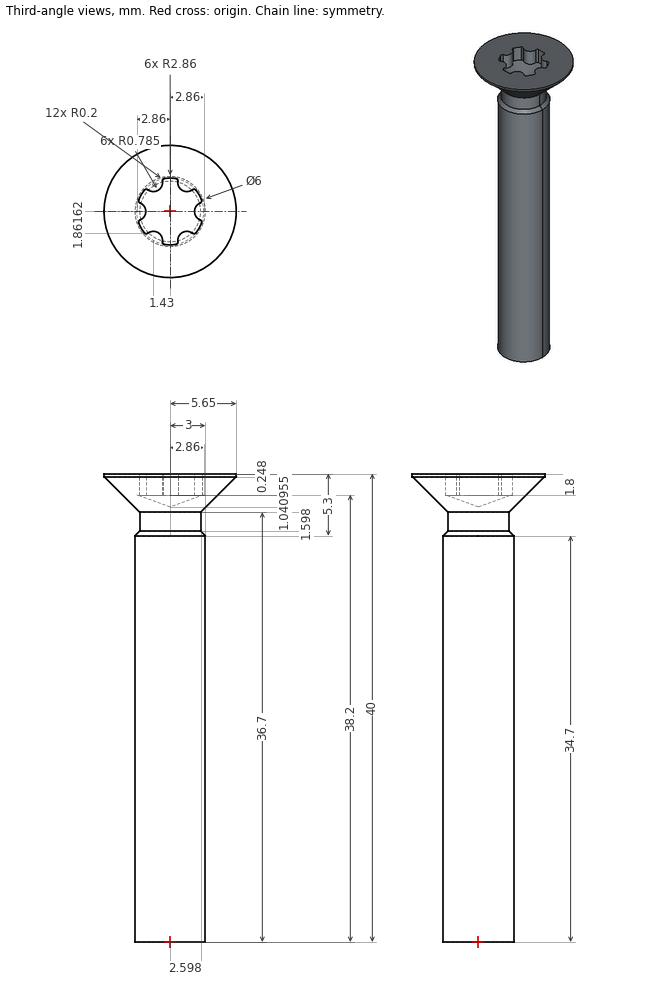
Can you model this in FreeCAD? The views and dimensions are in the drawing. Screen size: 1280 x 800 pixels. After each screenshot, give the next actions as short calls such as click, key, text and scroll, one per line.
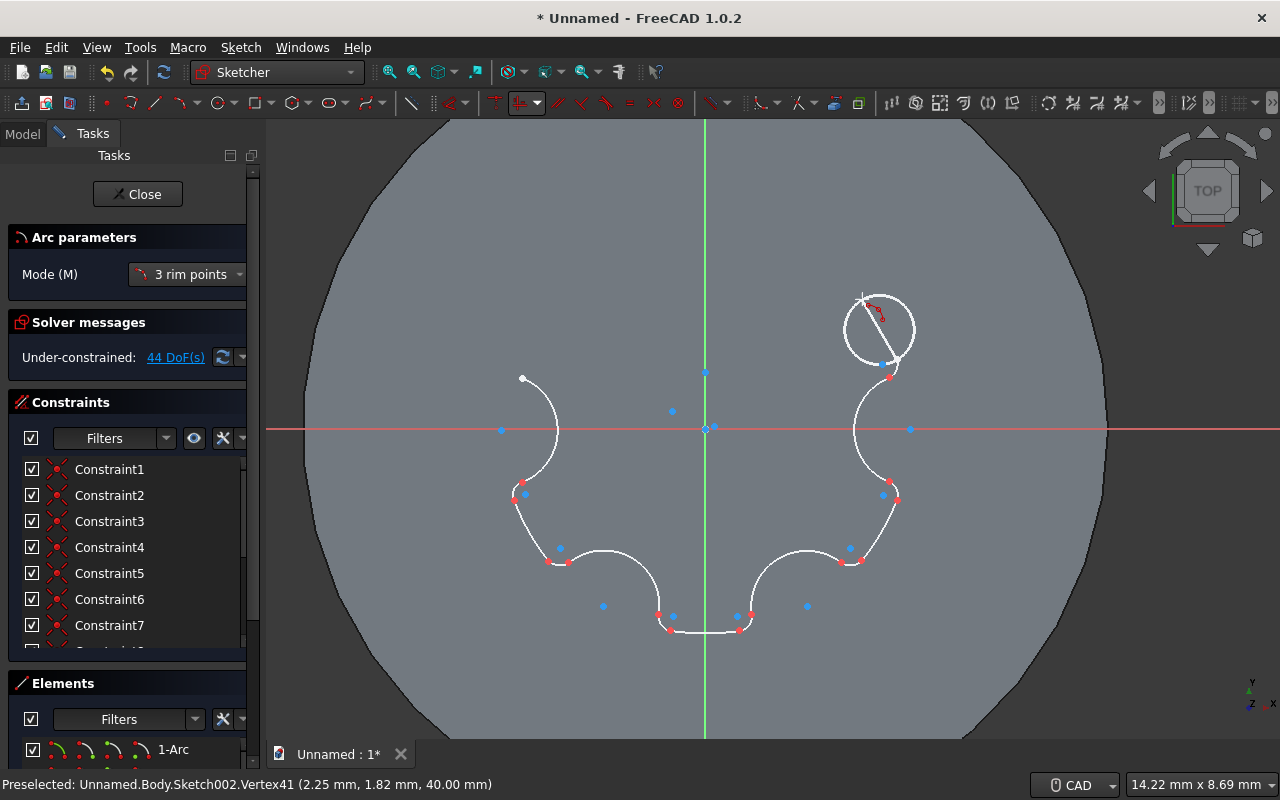
scroll(882, 327, up, 9)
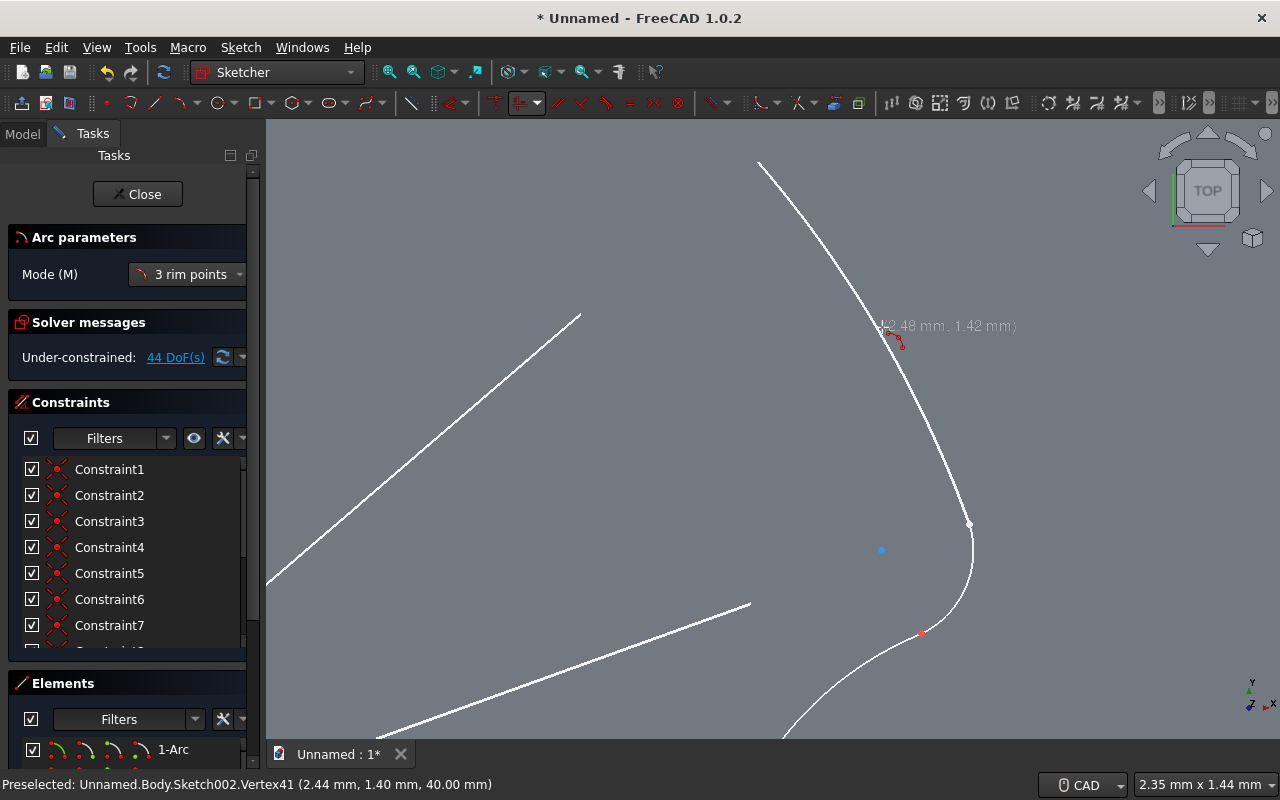
click(878, 327)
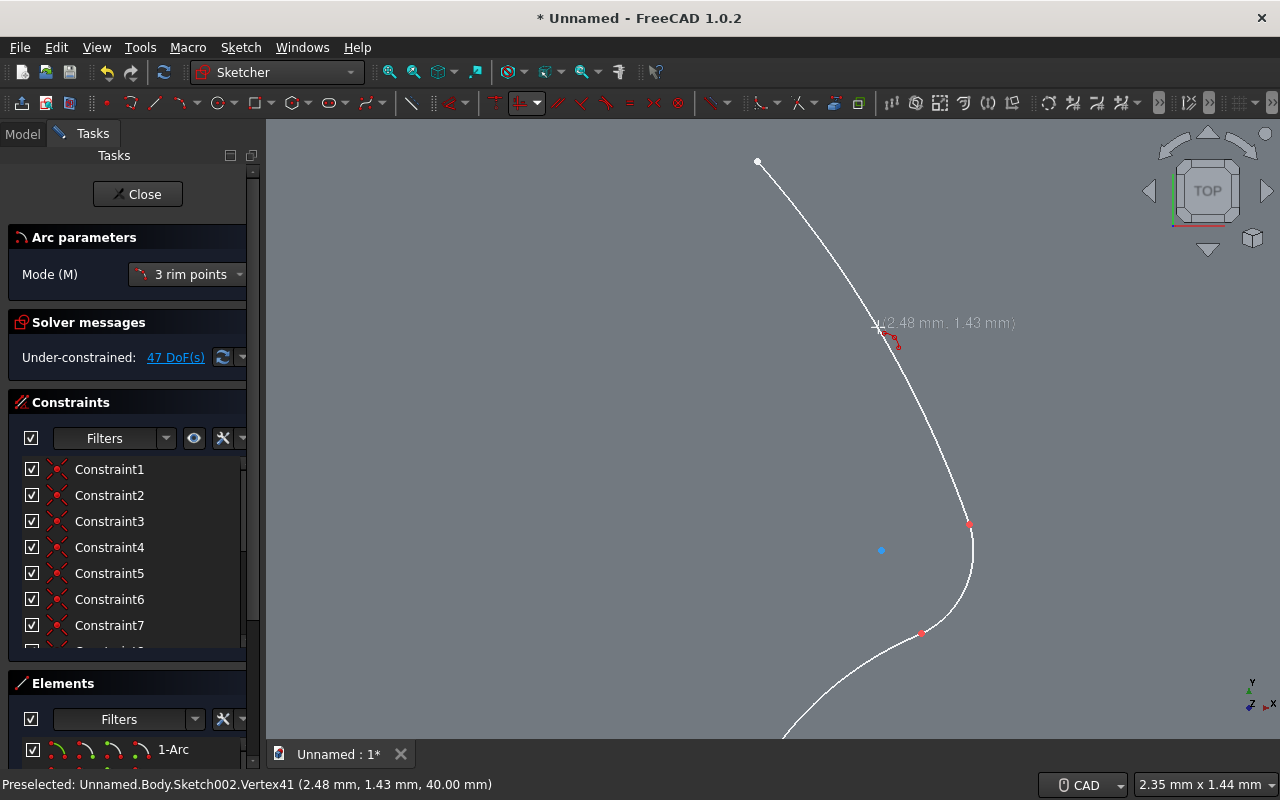
scroll(882, 327, down, 9)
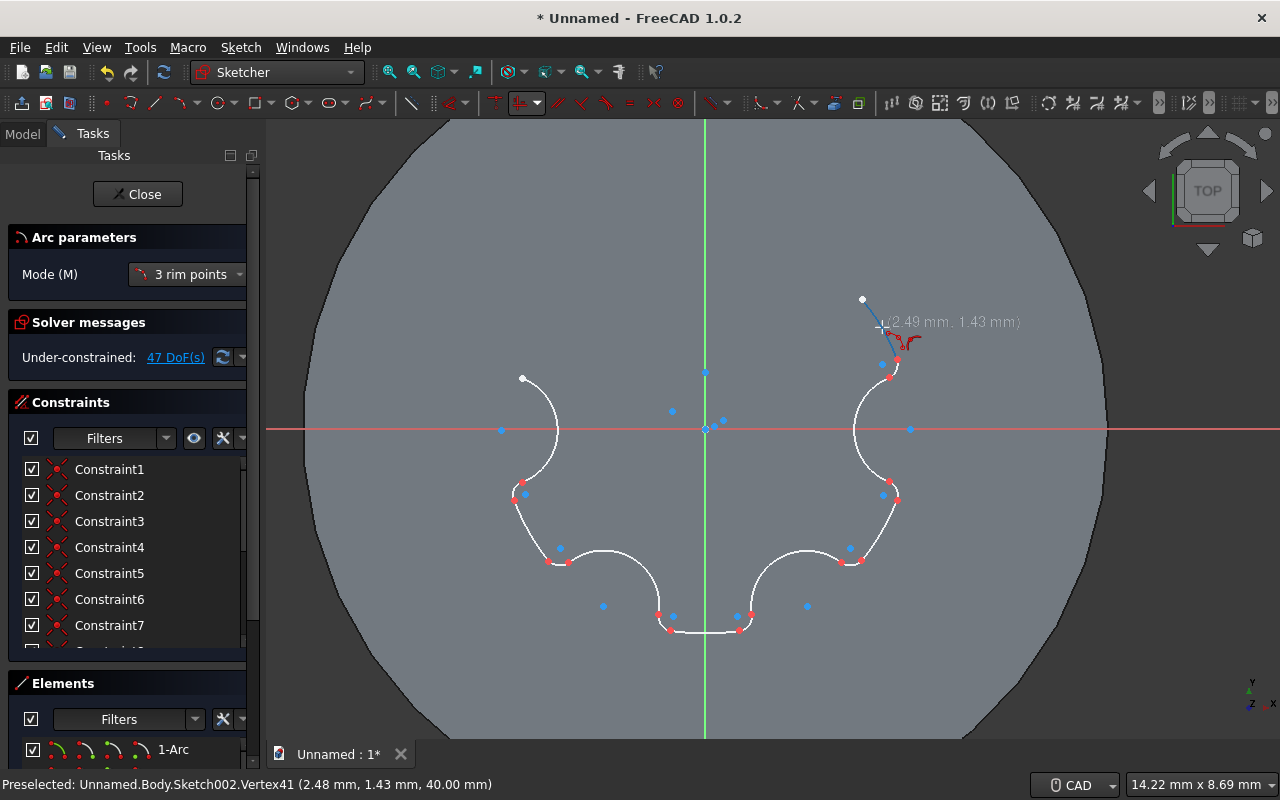
click(862, 300)
click(842, 297)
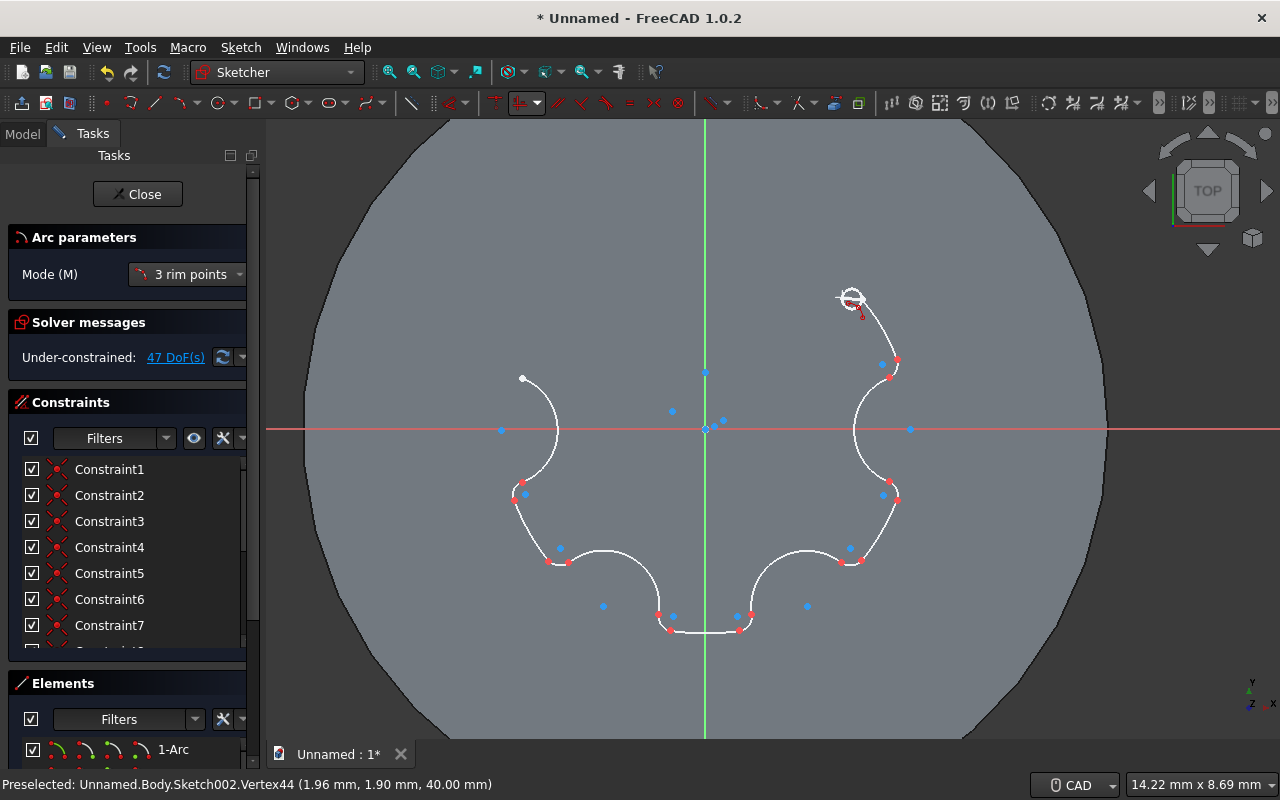
scroll(852, 294, up, 7)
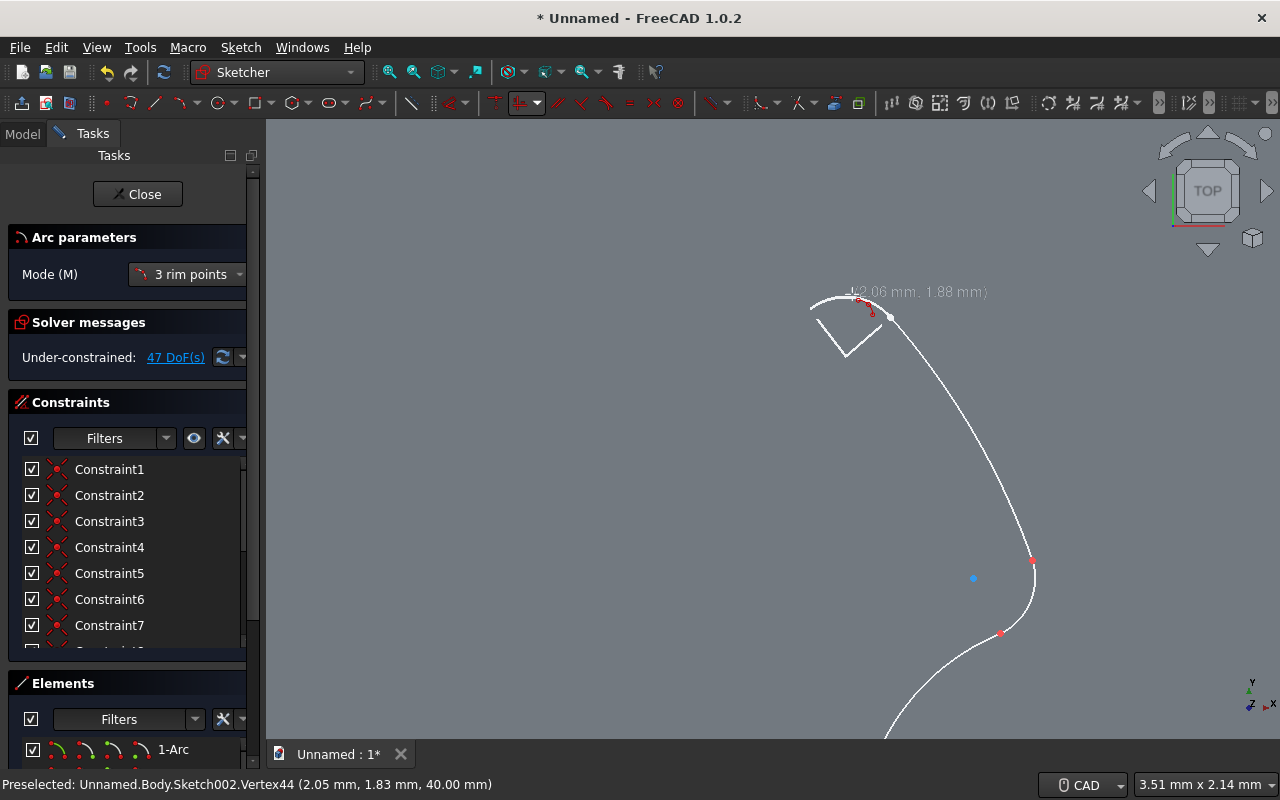
click(852, 291)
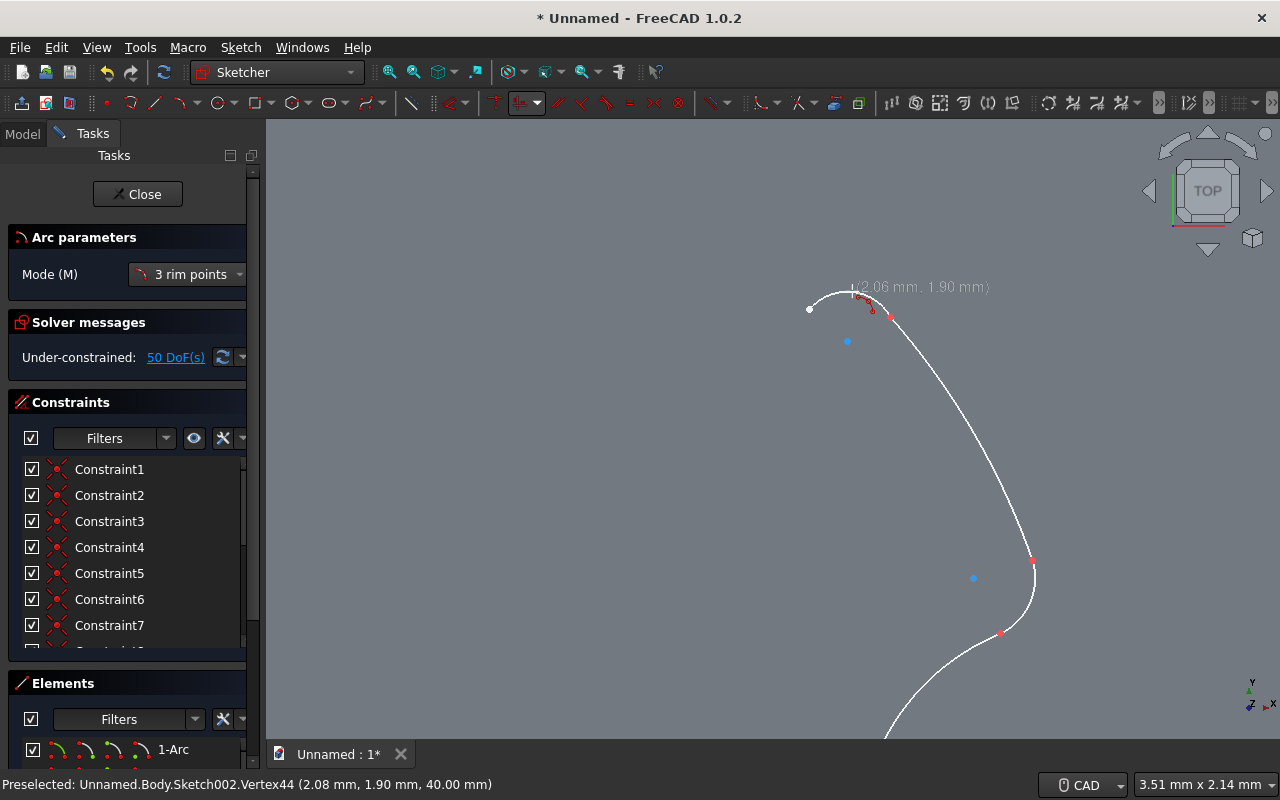
scroll(852, 294, down, 7)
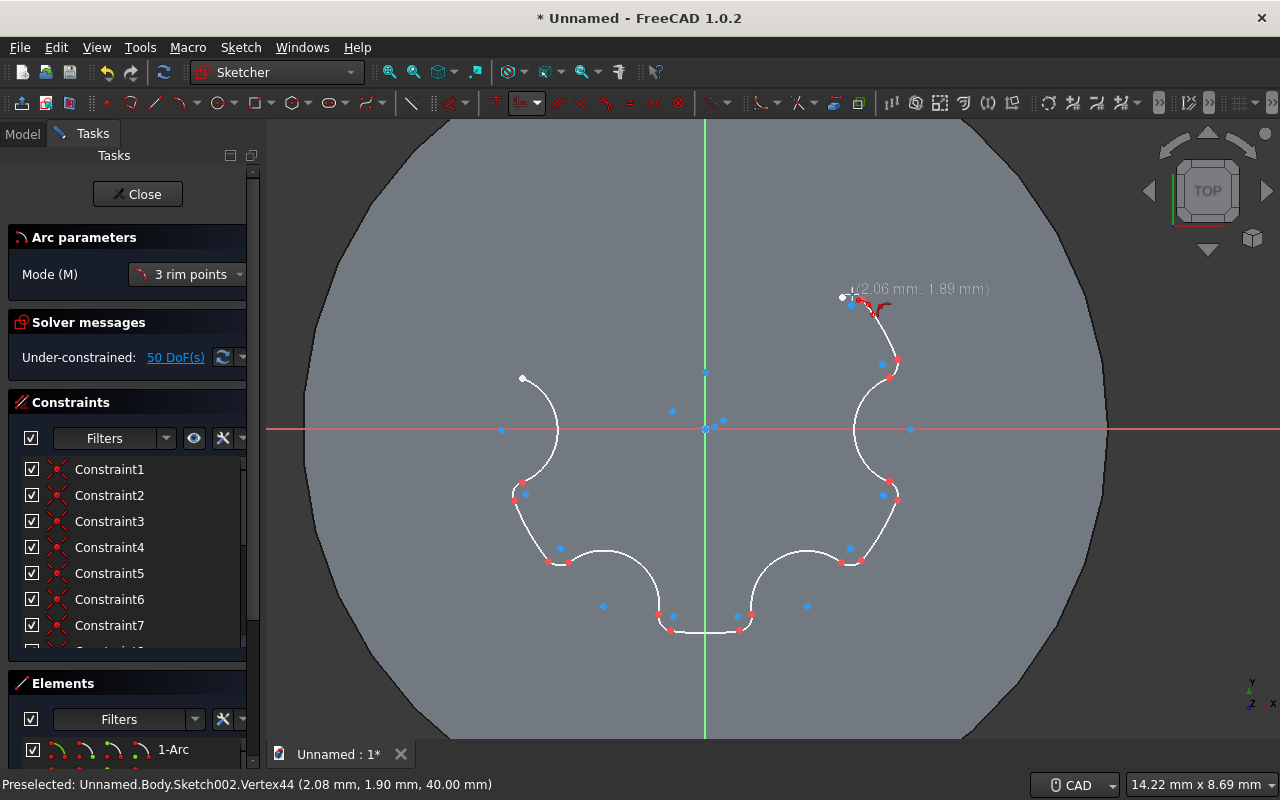
click(842, 298)
click(752, 244)
click(779, 301)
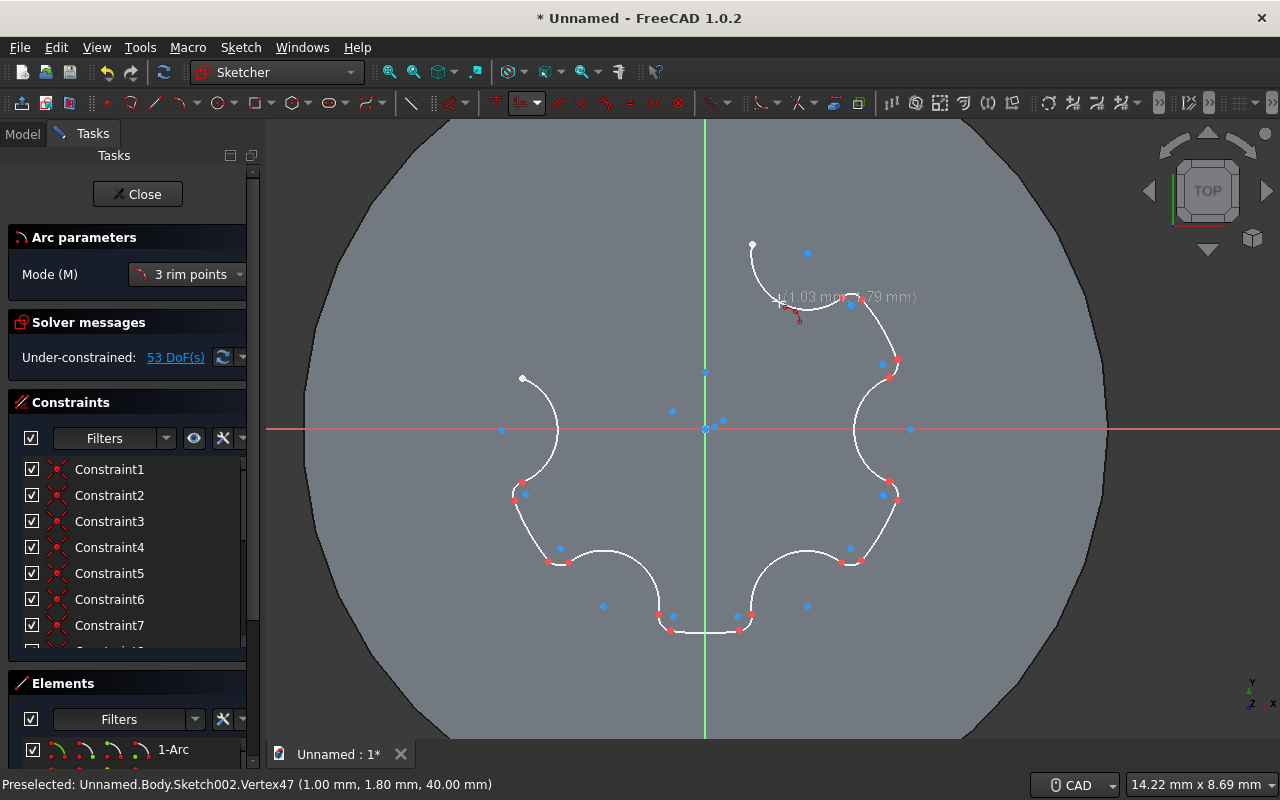
click(752, 245)
click(740, 228)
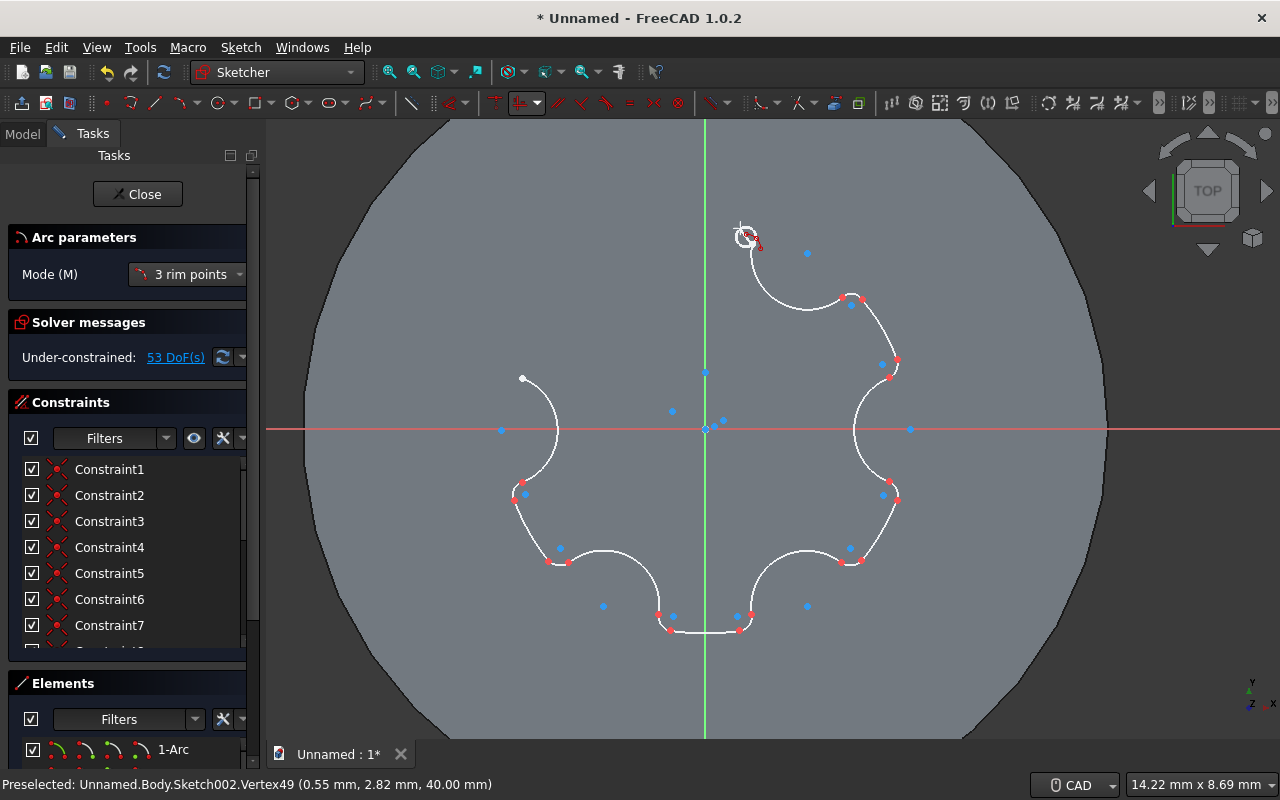
scroll(749, 234, up, 7)